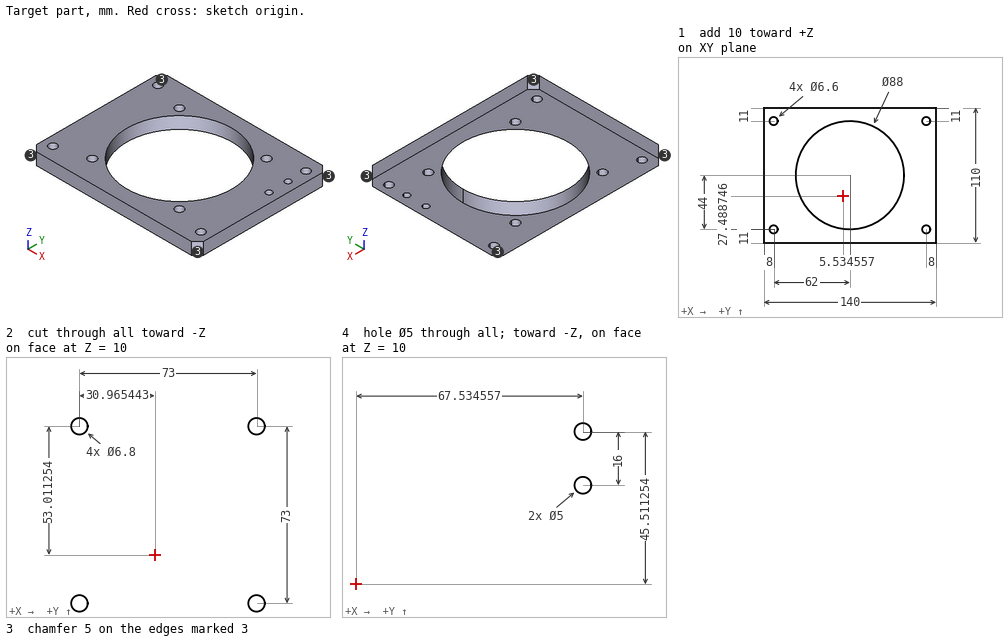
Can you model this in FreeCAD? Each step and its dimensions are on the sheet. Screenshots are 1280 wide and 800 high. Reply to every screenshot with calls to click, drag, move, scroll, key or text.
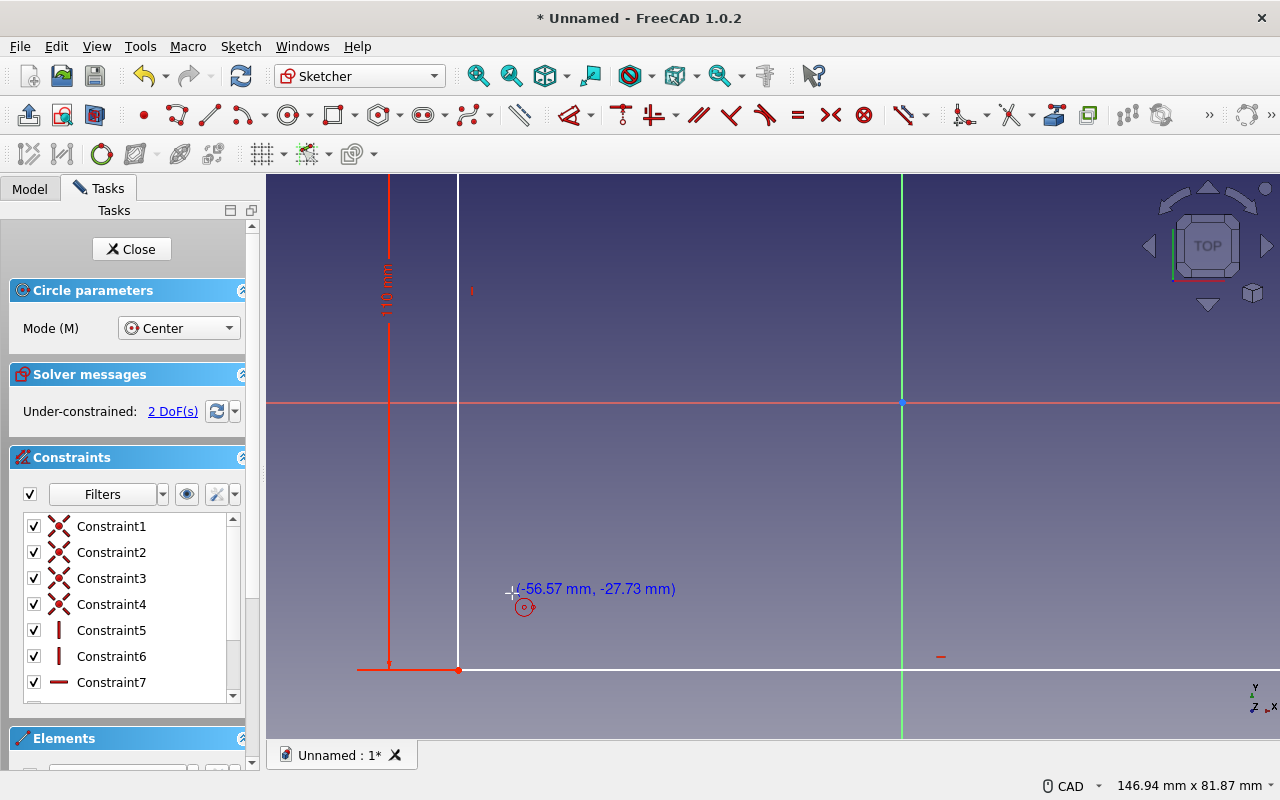
click(512, 593)
move(529, 577)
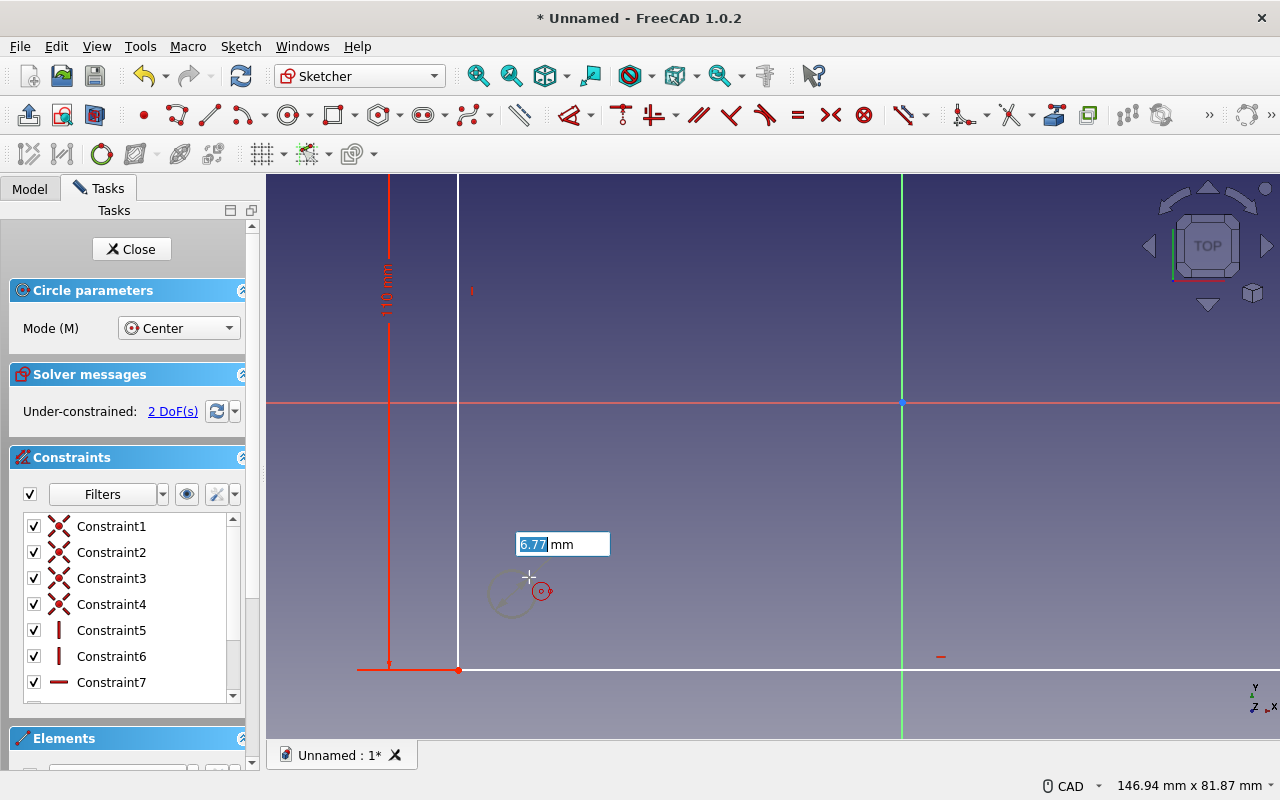
text(6.6)
key(Return)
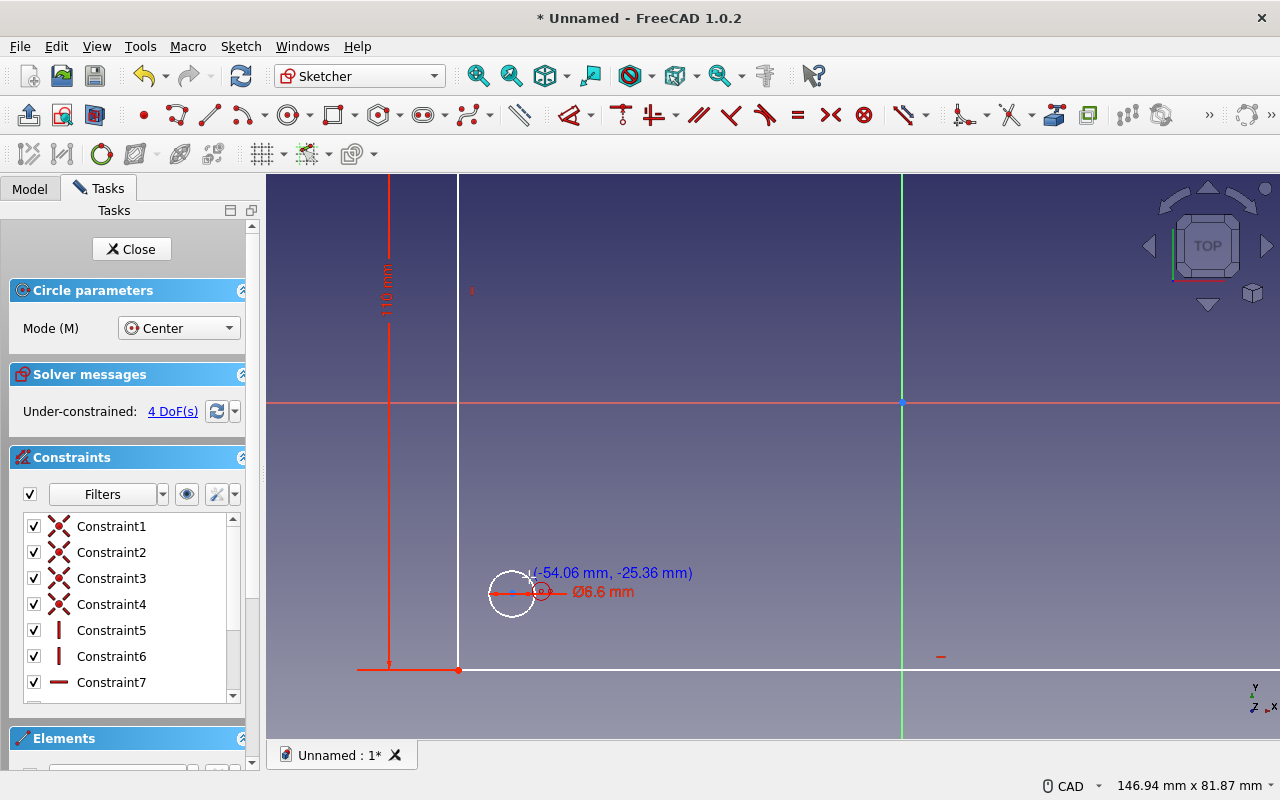
scroll(512, 593, down, 4)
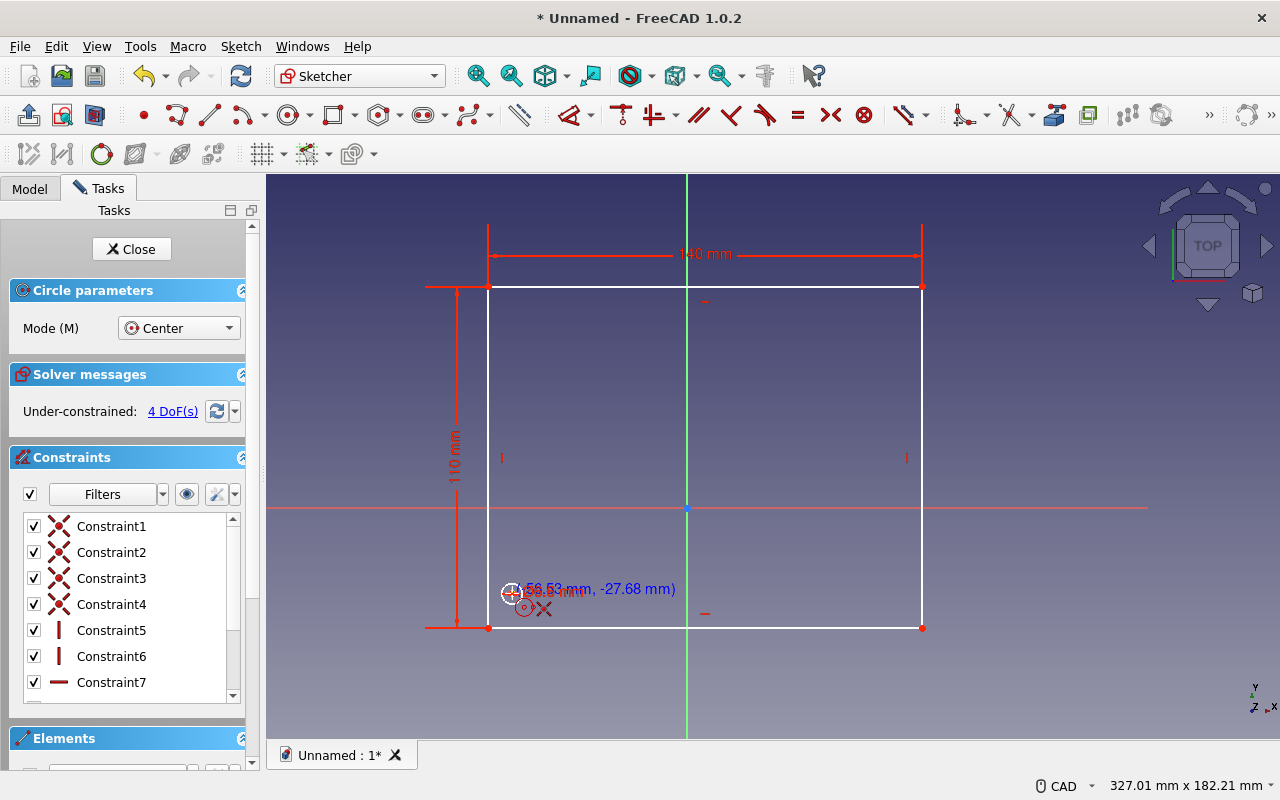
scroll(897, 593, up, 4)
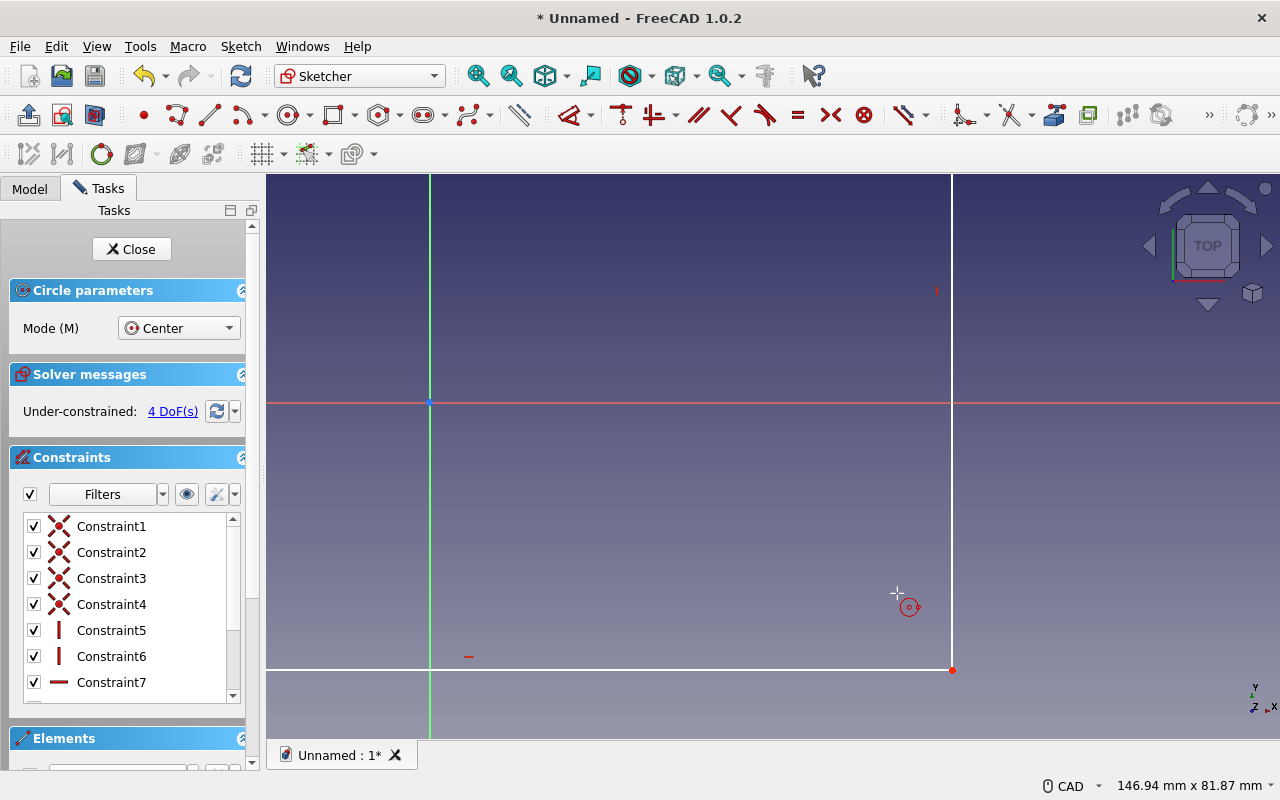
click(896, 593)
move(912, 577)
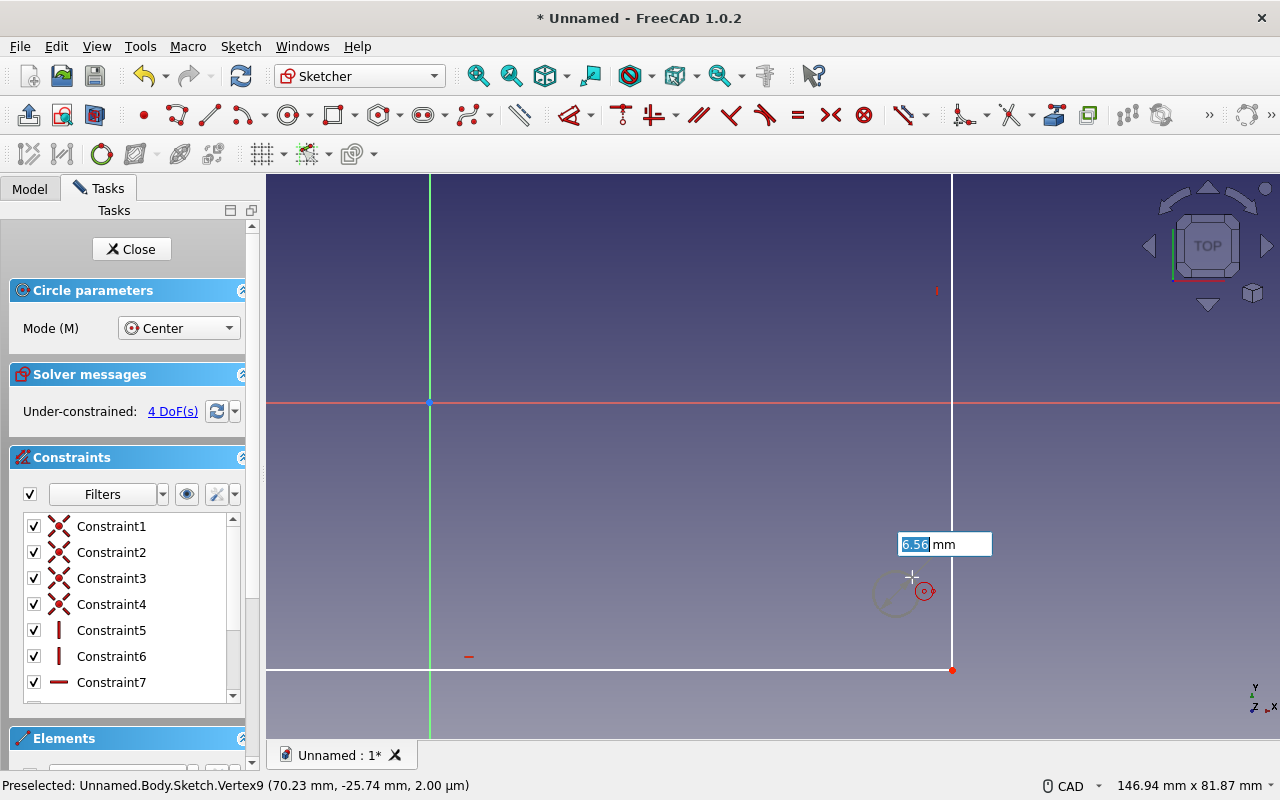
text(6.6)
key(Return)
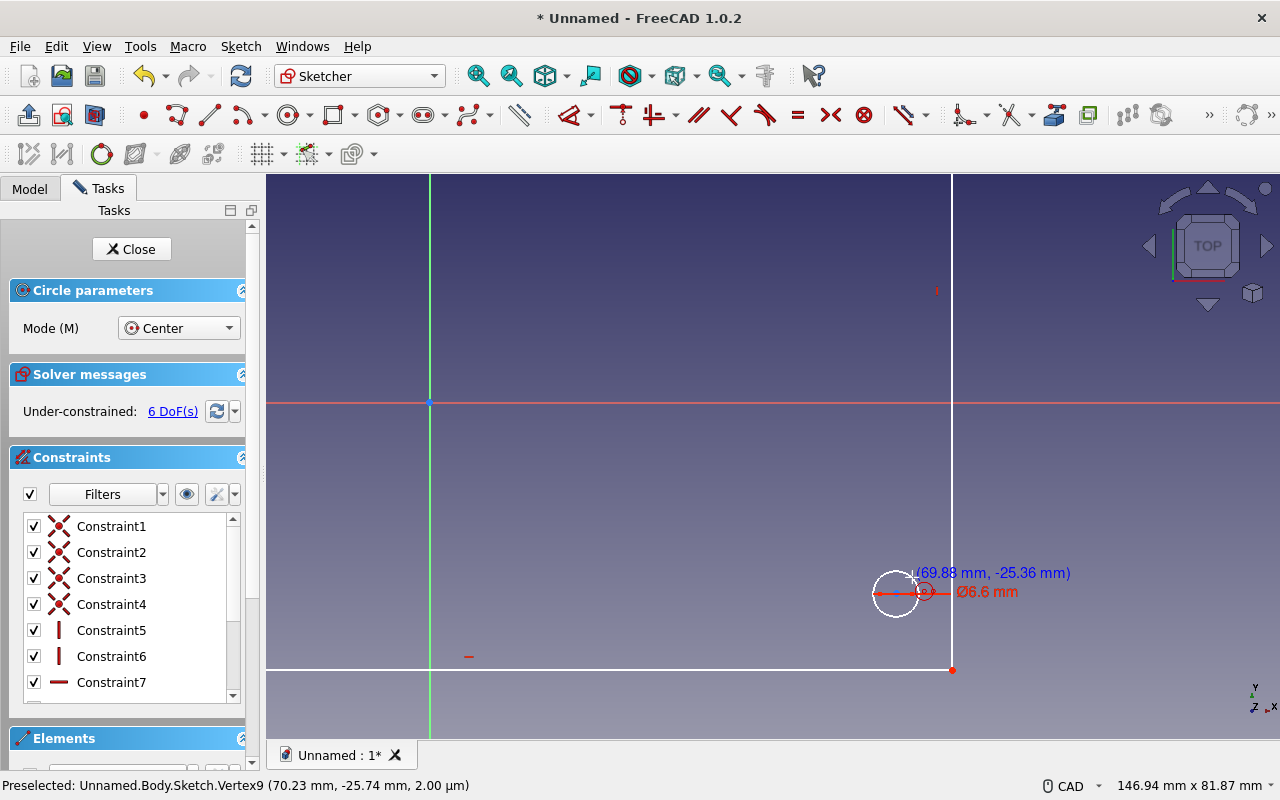
click(468, 289)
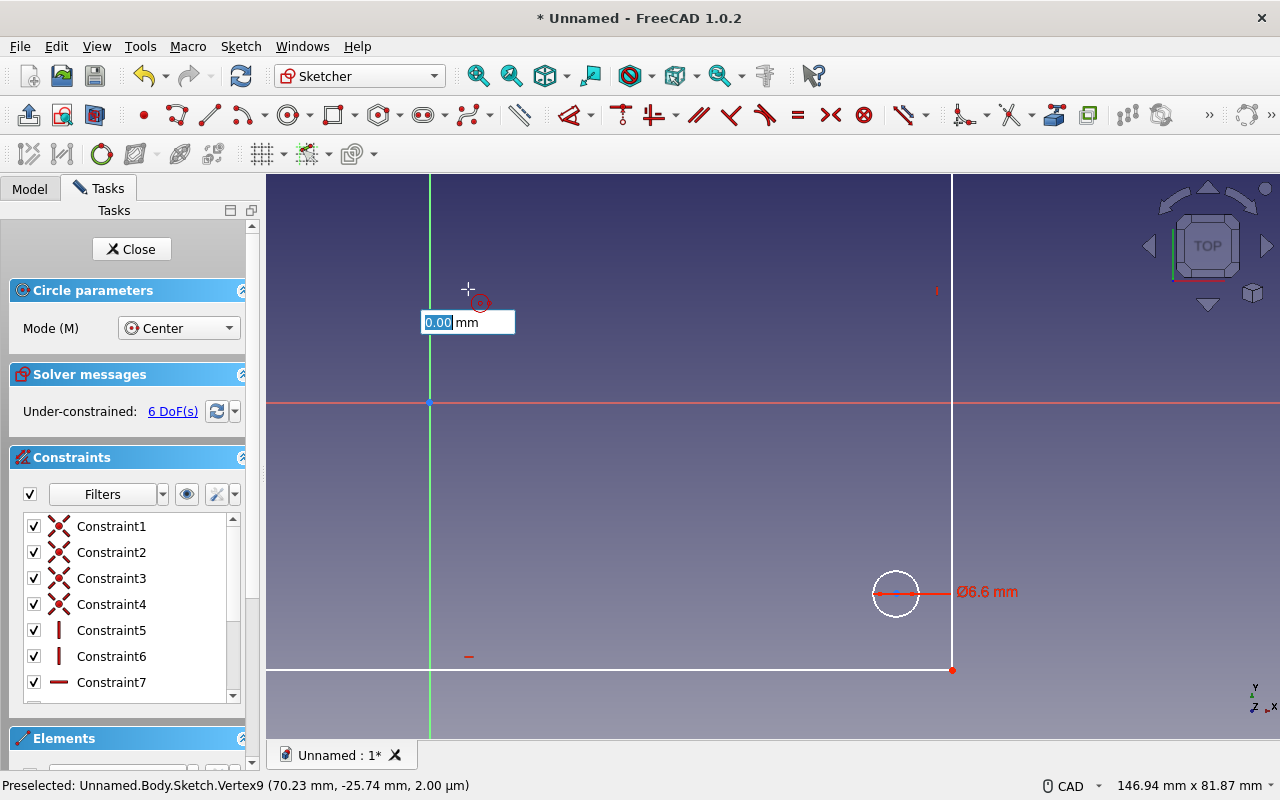
scroll(897, 593, down, 4)
move(801, 360)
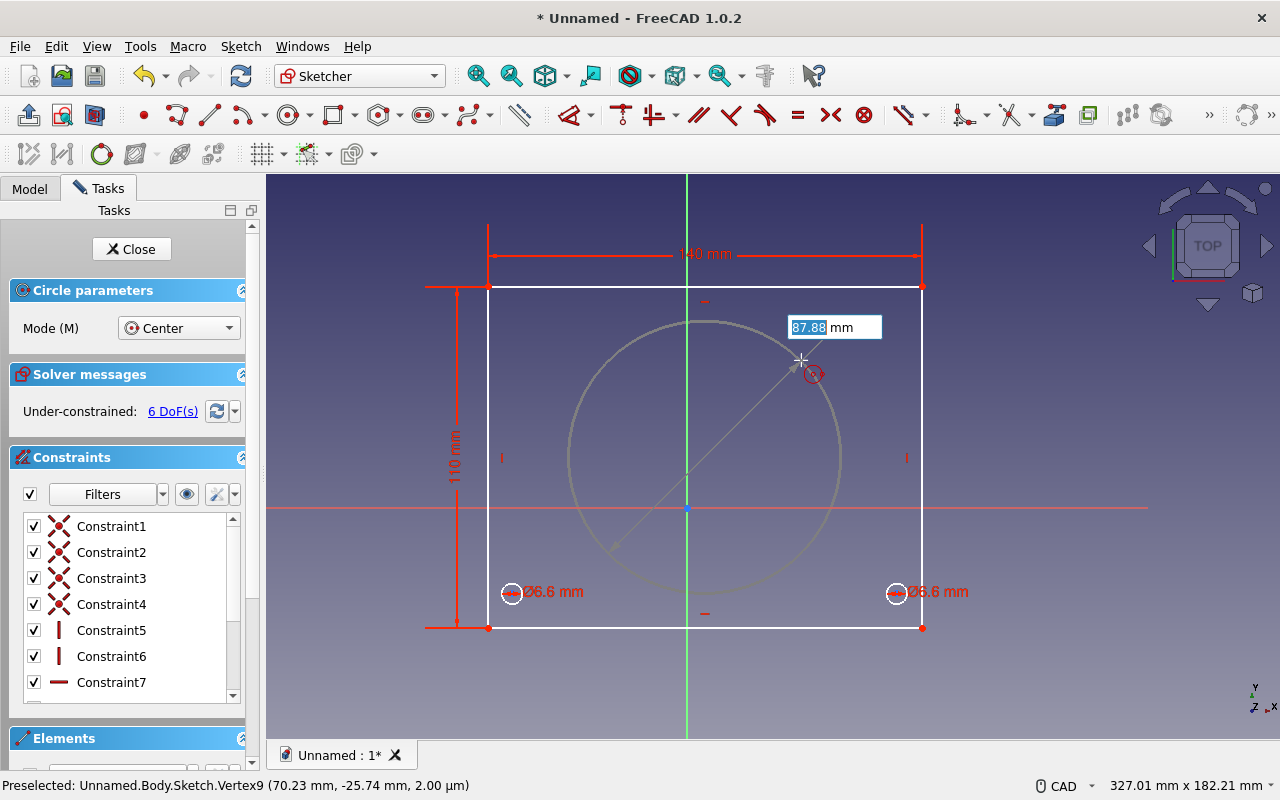
text(88)
key(Return)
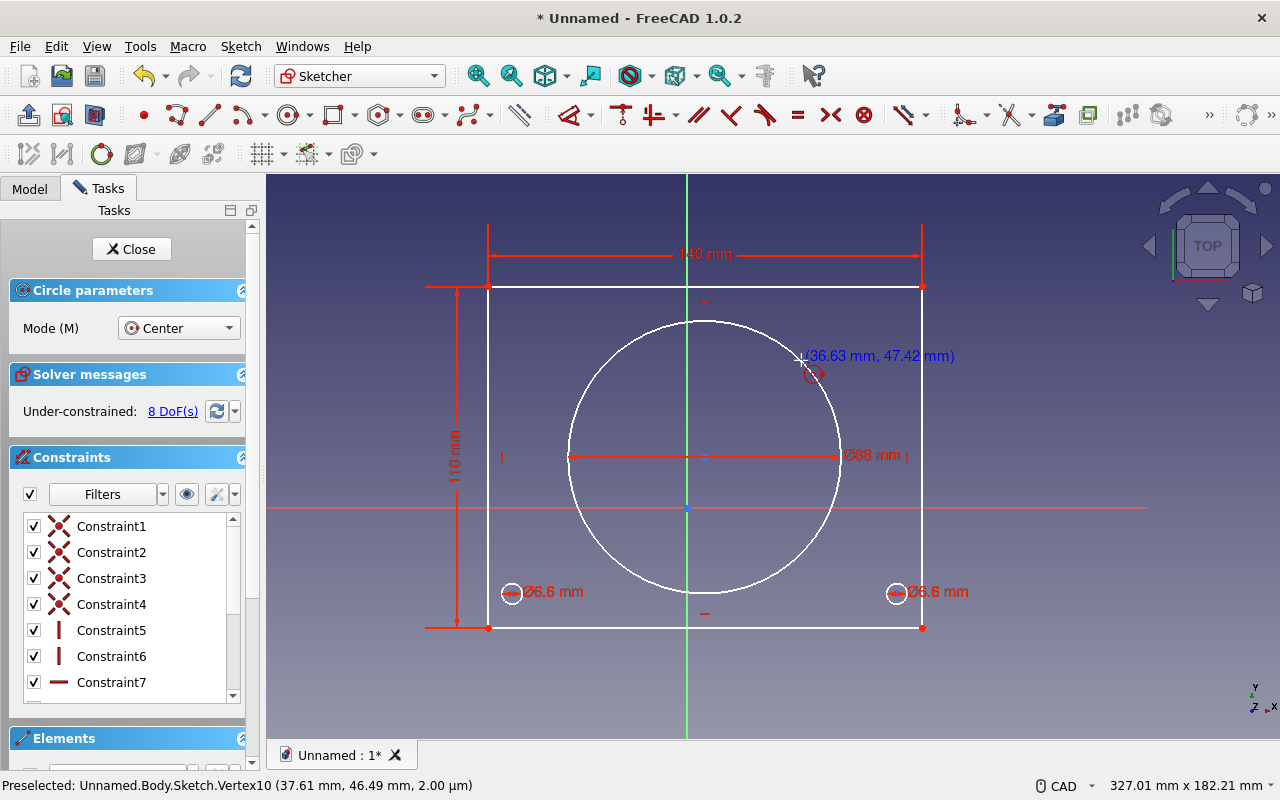
scroll(512, 320, up, 4)